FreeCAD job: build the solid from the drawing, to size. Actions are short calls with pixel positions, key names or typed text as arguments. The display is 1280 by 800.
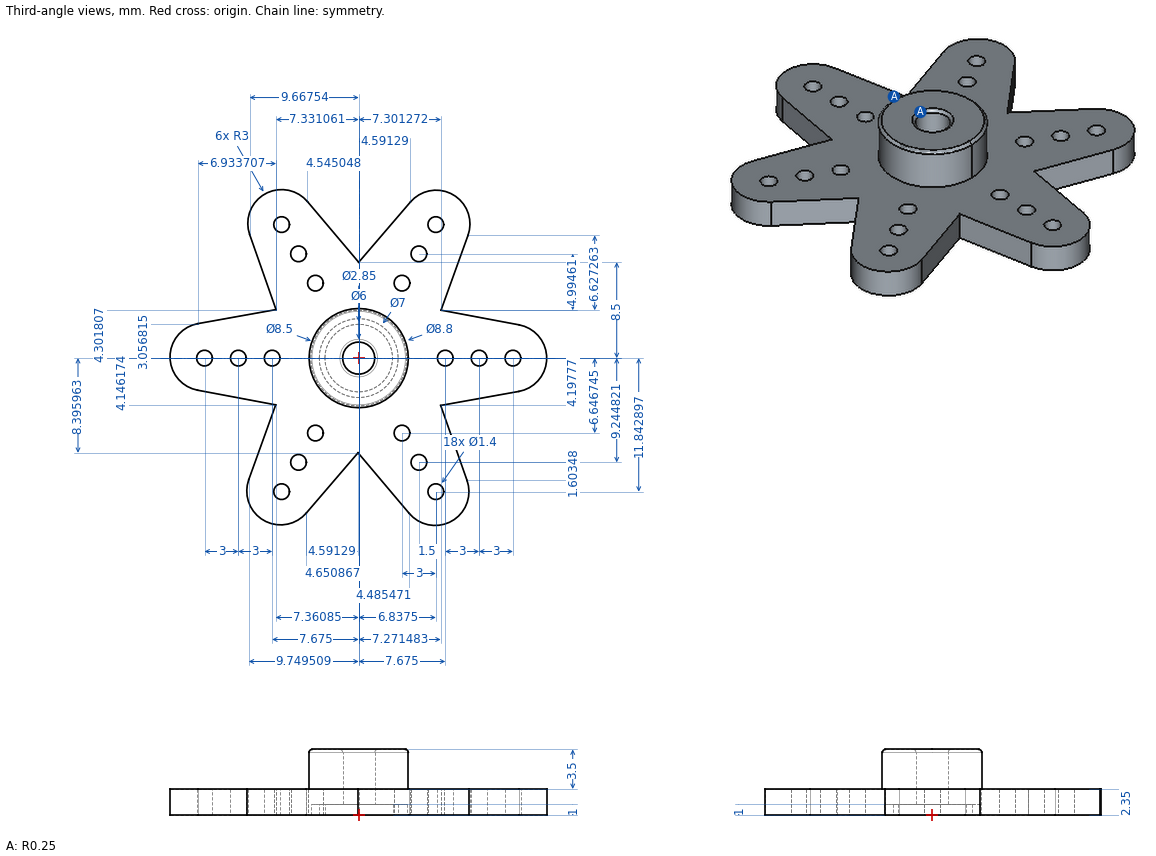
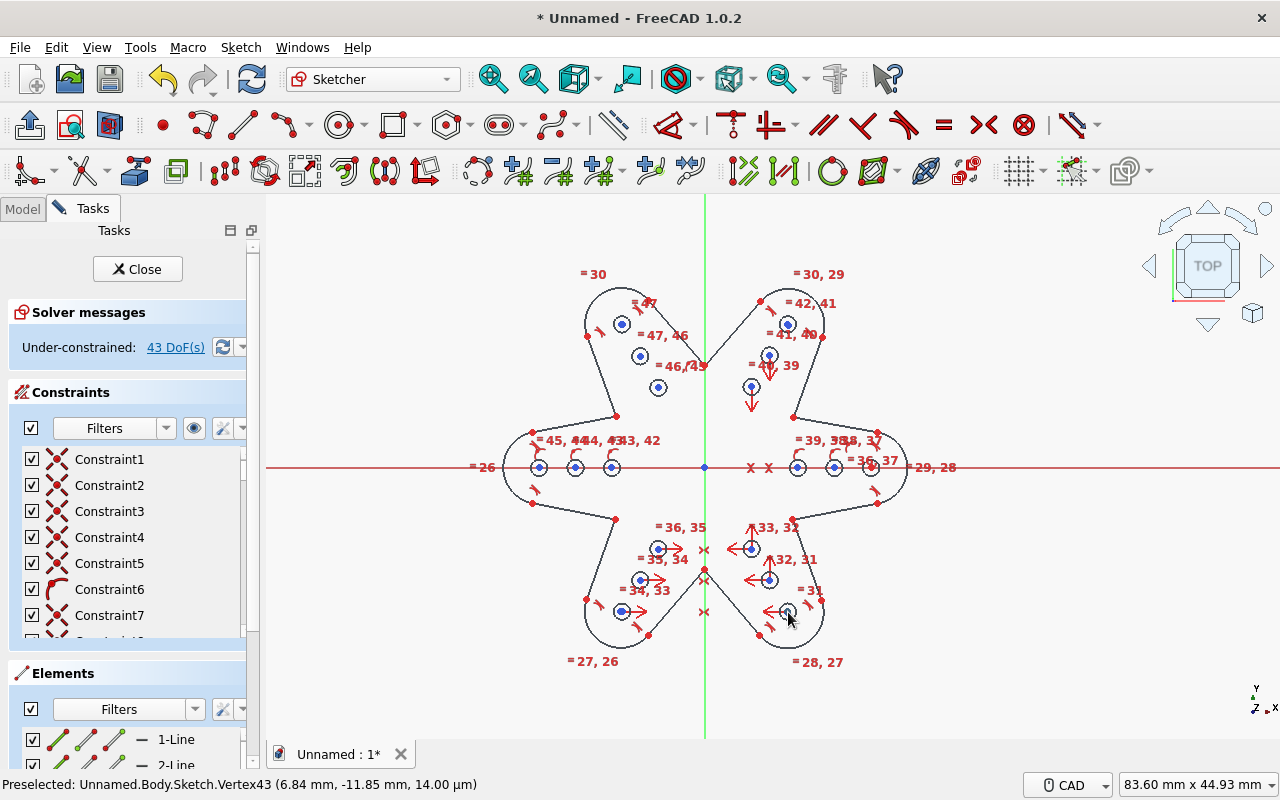
scroll(788, 324, up, 14)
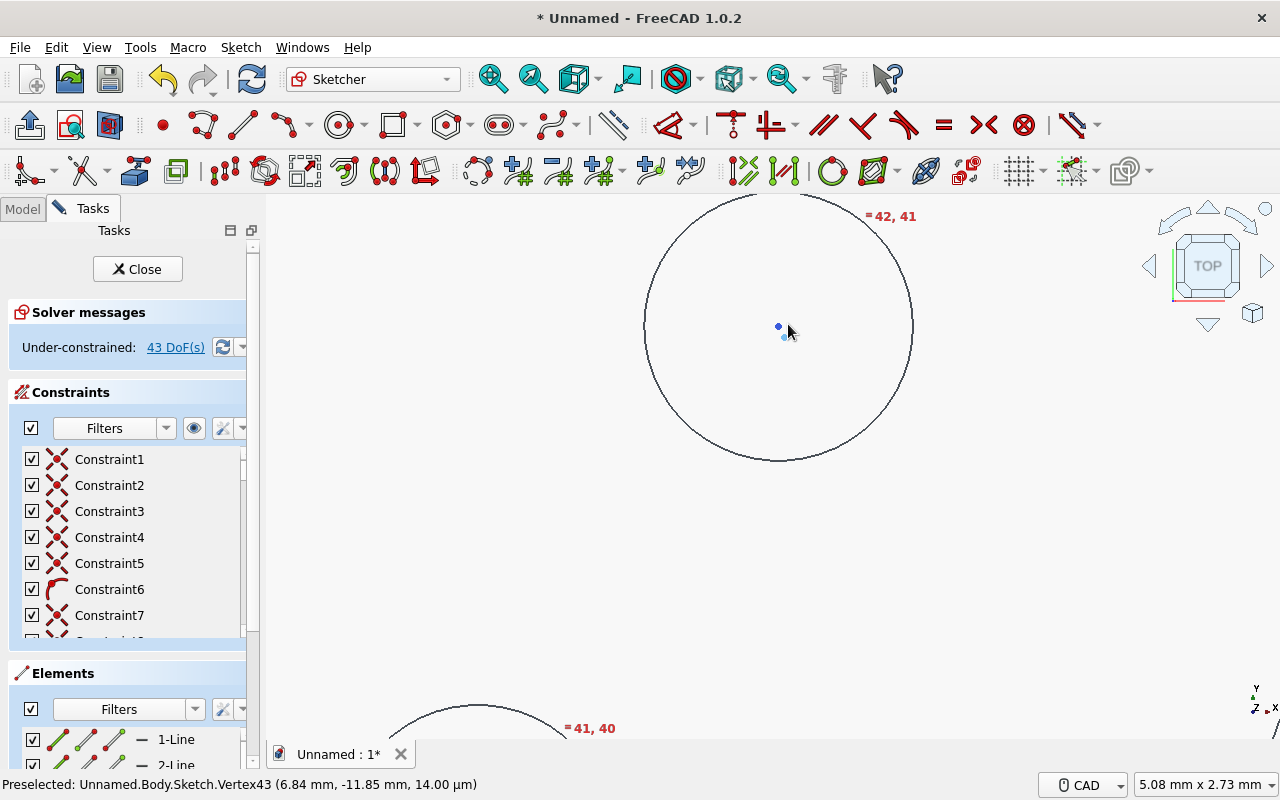
click(779, 326)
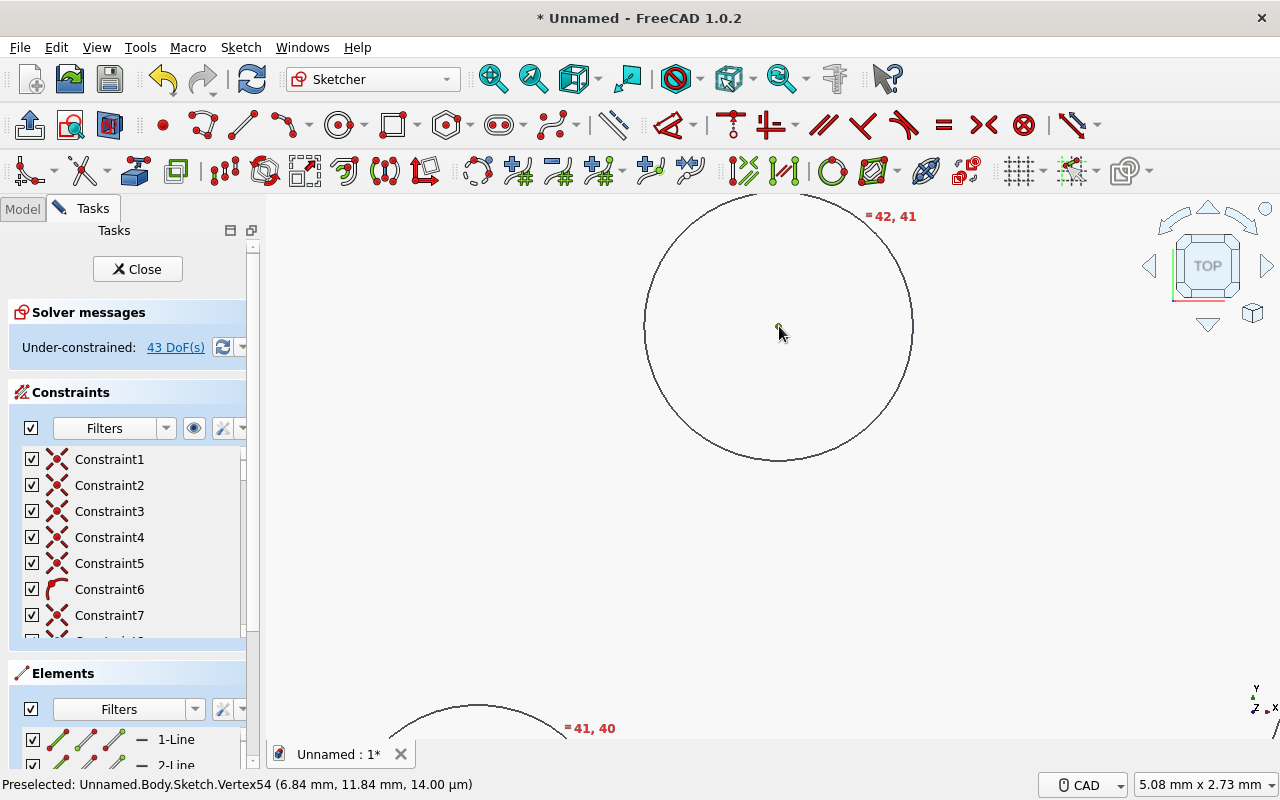
scroll(788, 323, down, 14)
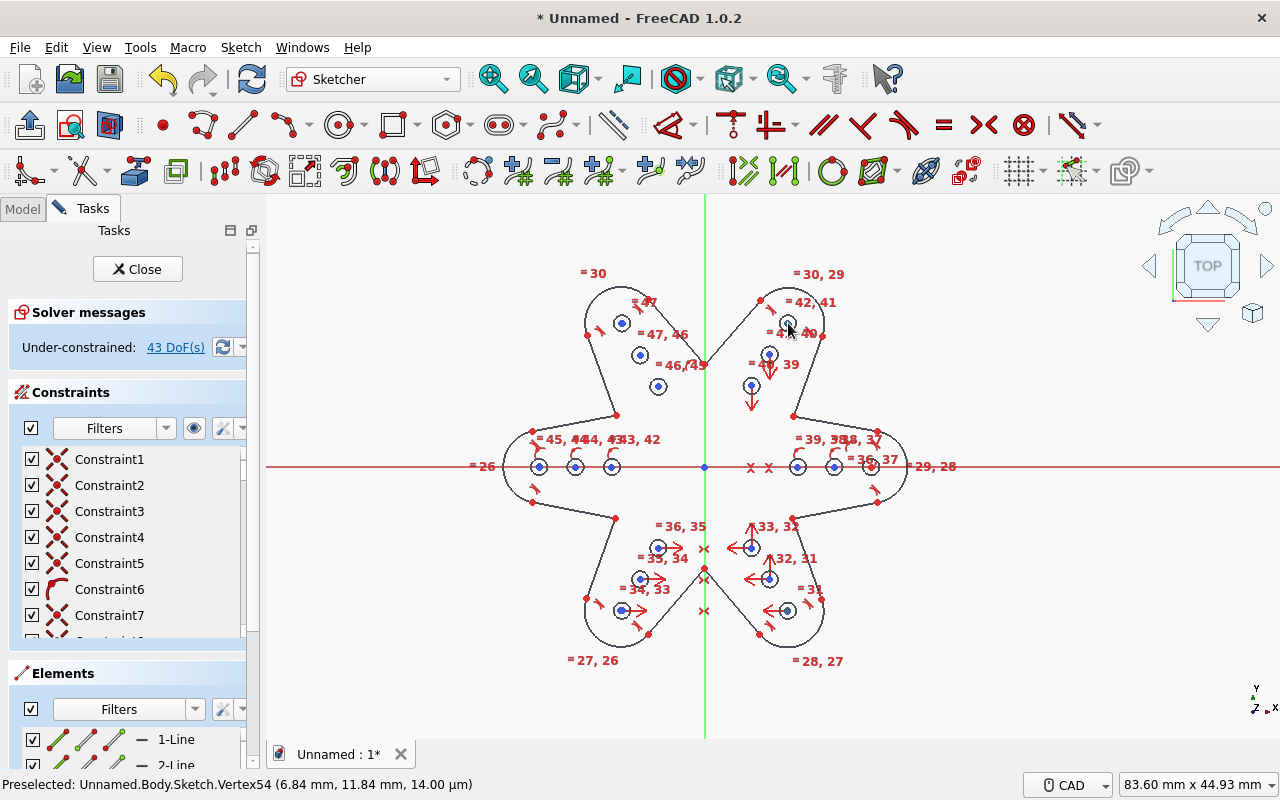
click(353, 467)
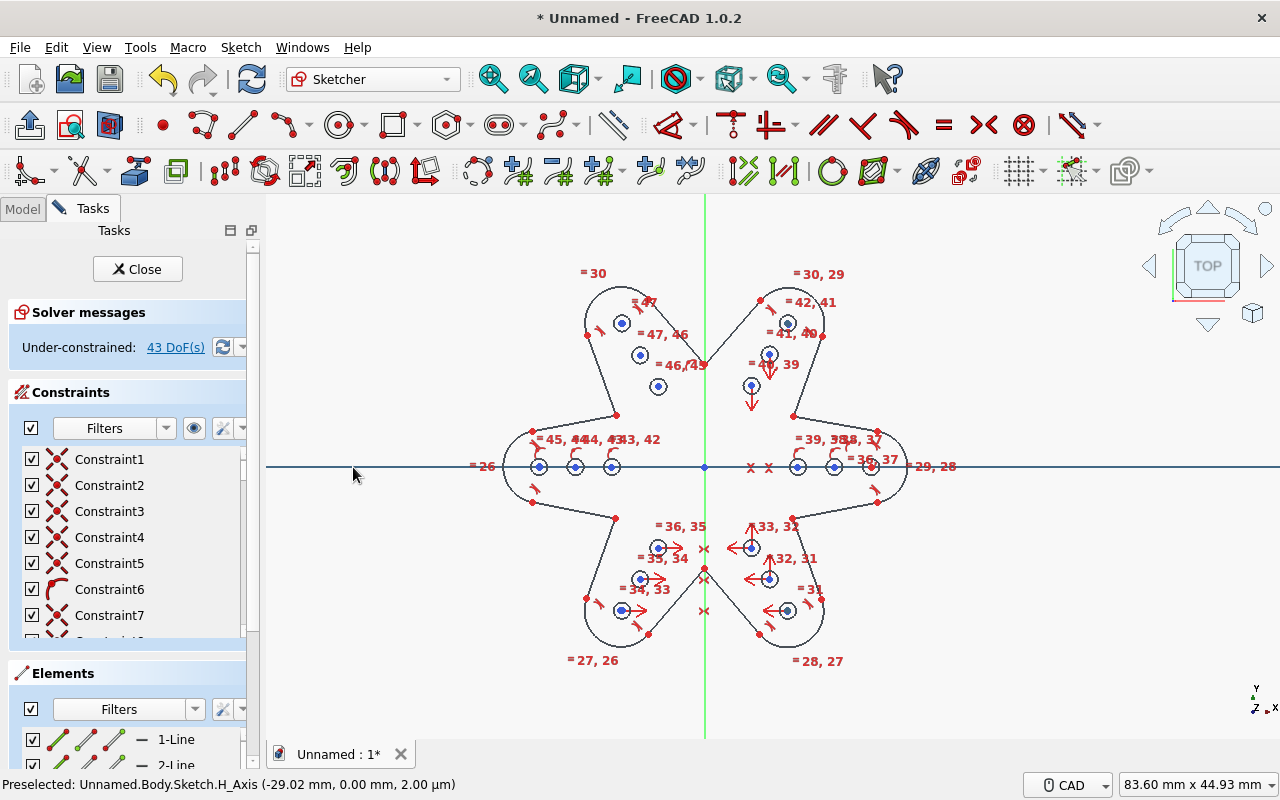
click(984, 126)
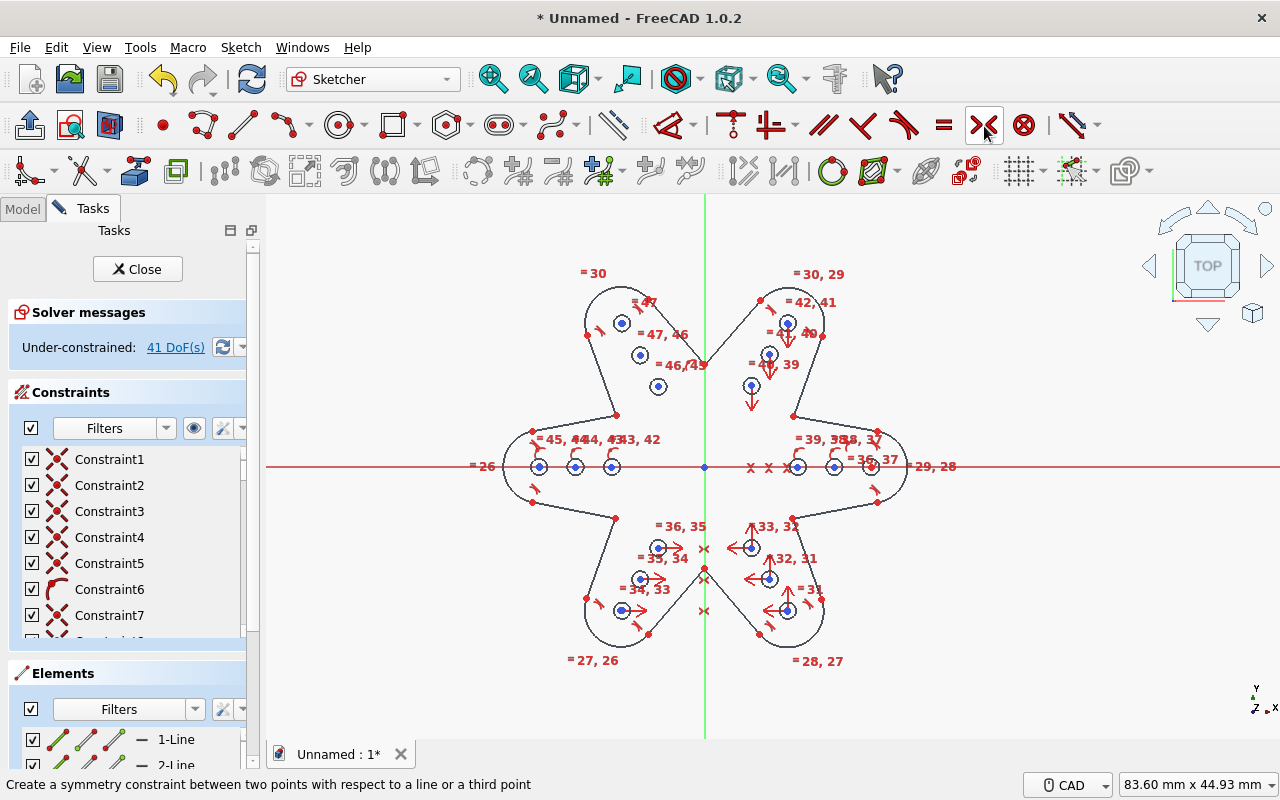
click(658, 548)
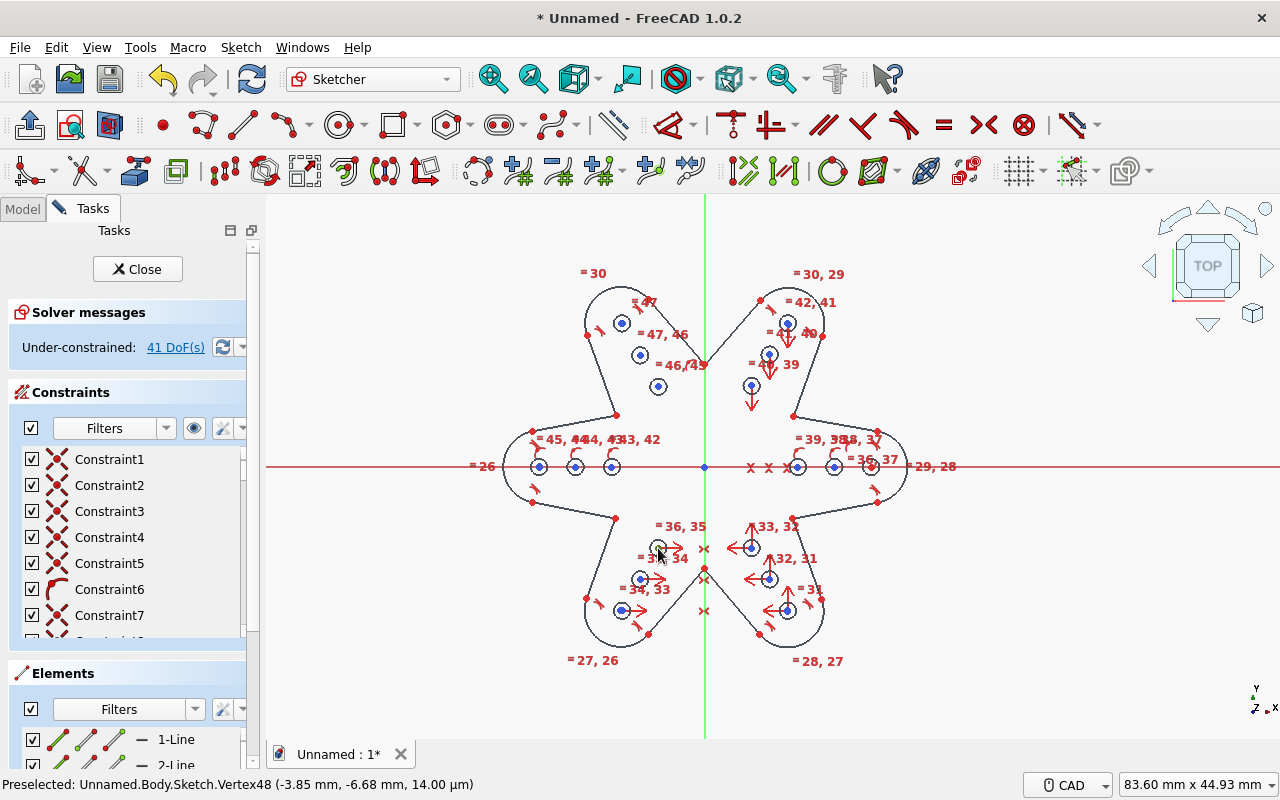
click(658, 387)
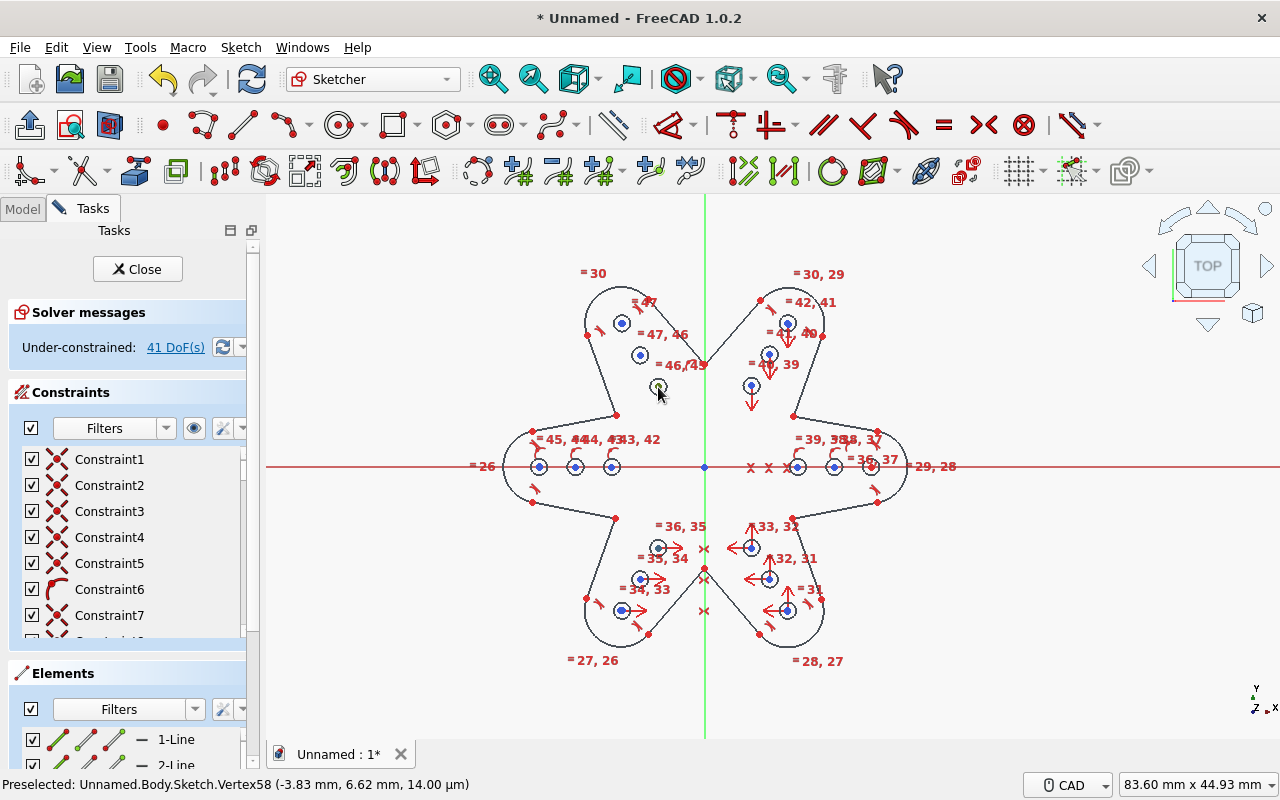
click(353, 467)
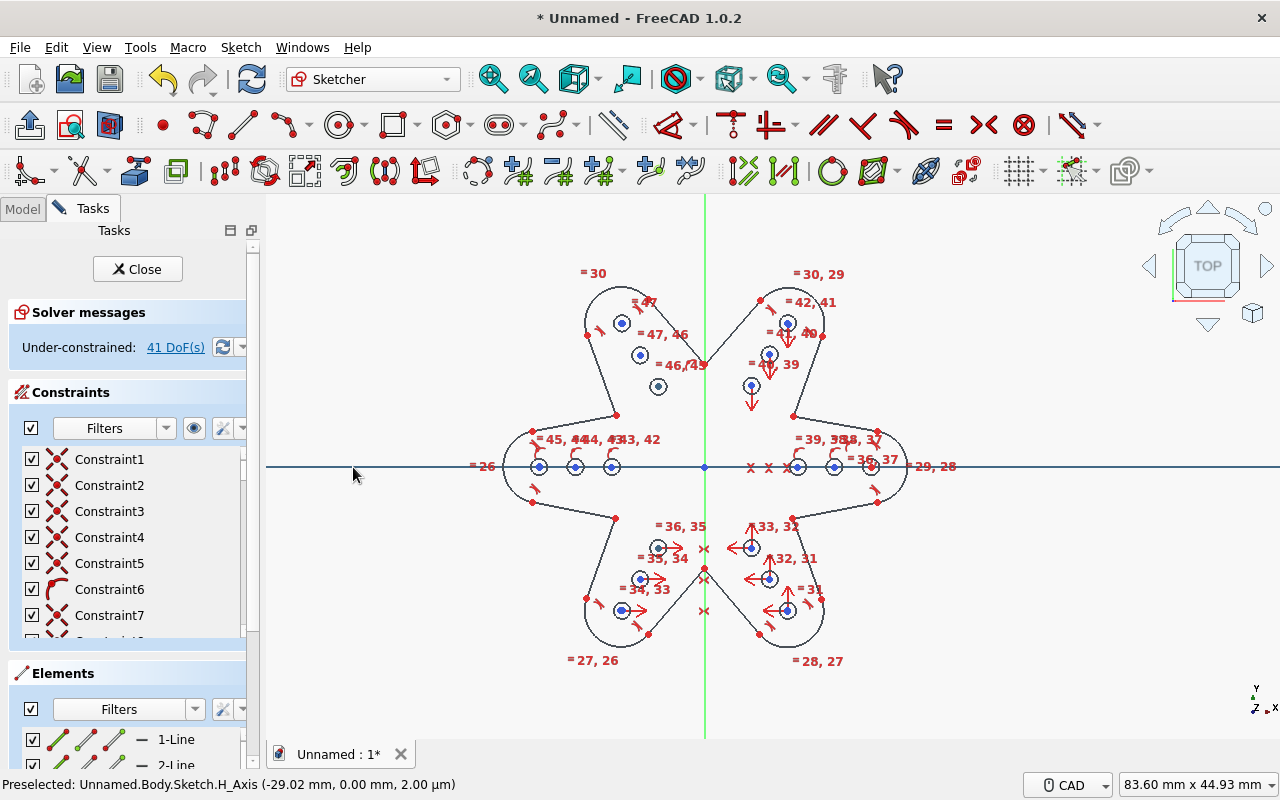
click(984, 126)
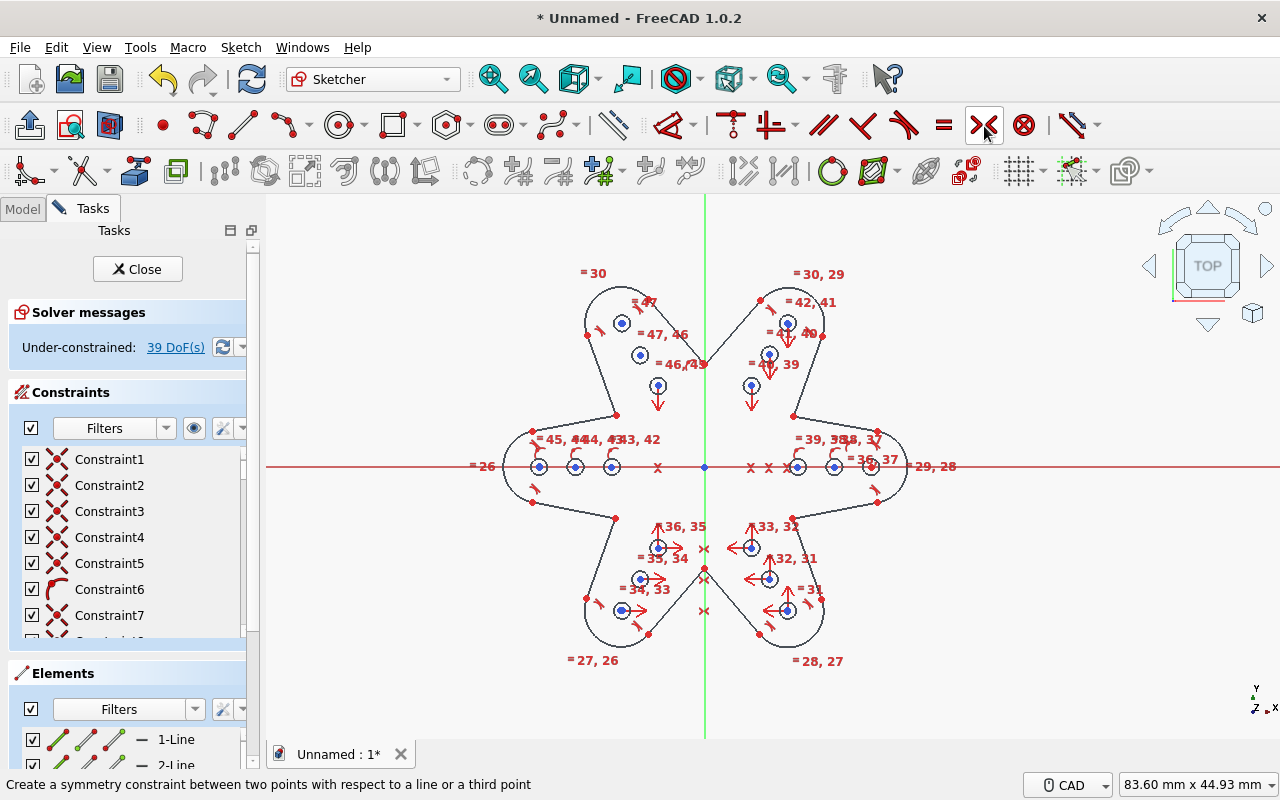
click(640, 579)